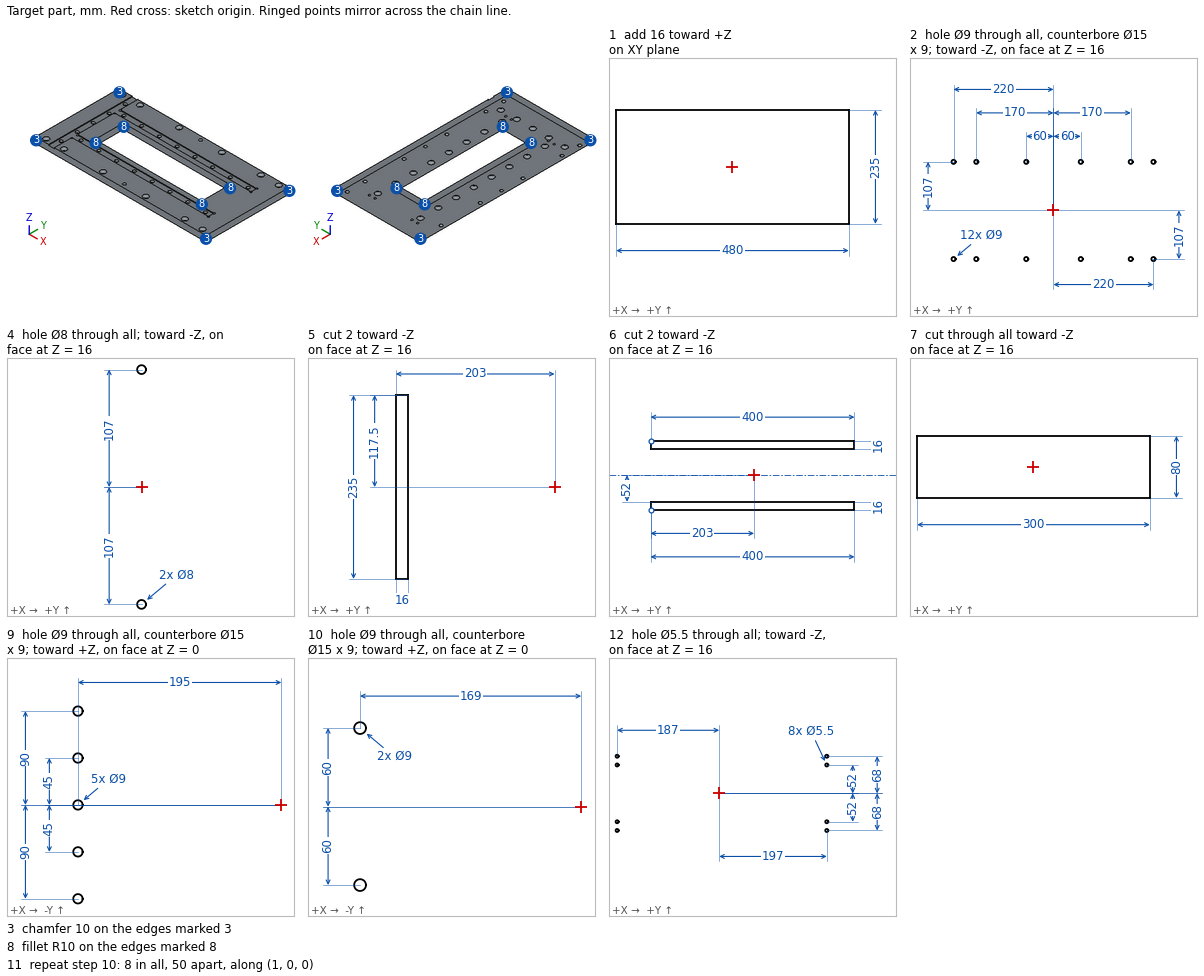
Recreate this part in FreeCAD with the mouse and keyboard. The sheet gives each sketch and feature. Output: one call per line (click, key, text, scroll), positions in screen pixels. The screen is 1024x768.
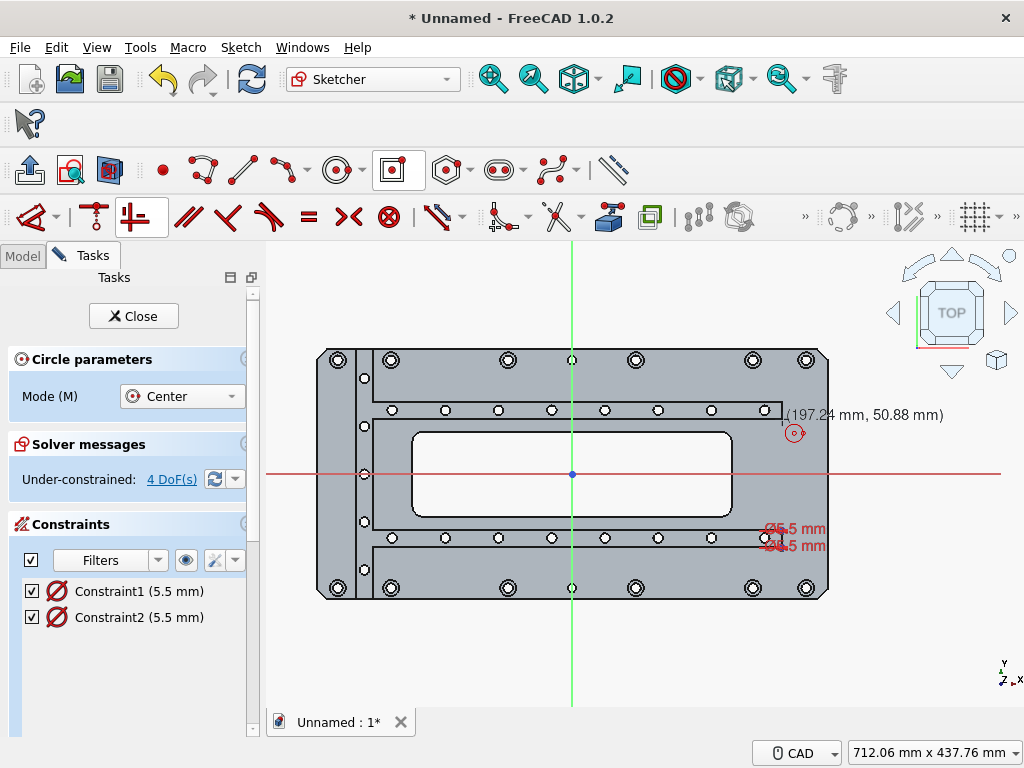
click(782, 419)
move(784, 417)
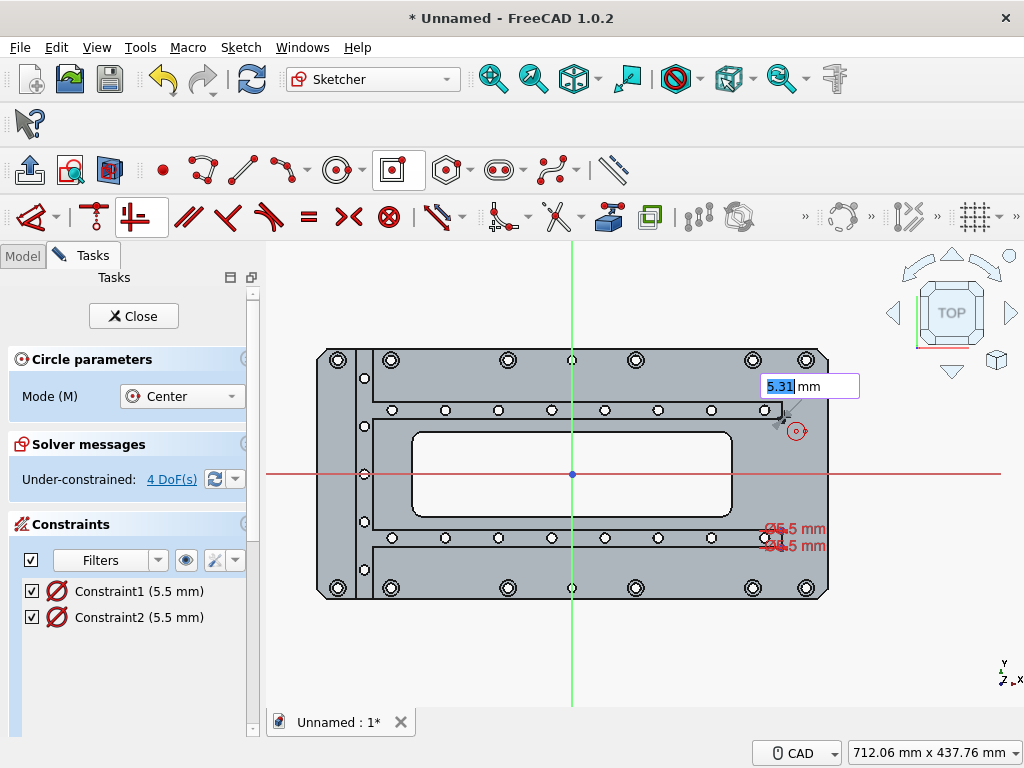
text(5.5)
key(Return)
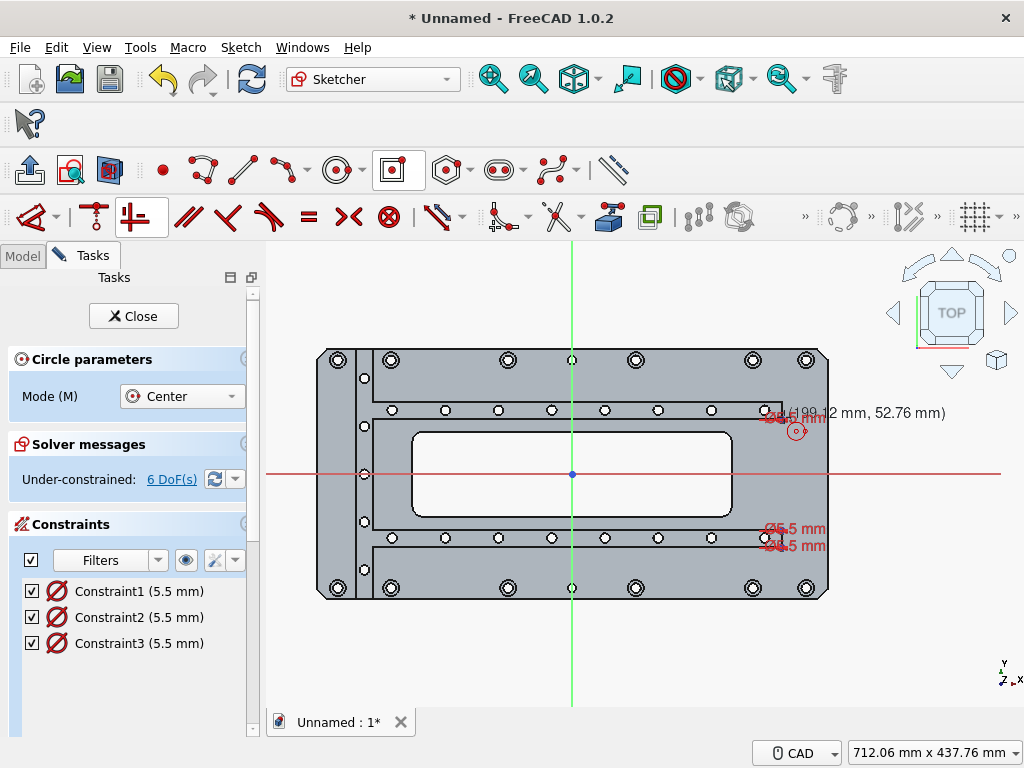
scroll(782, 402, up, 11)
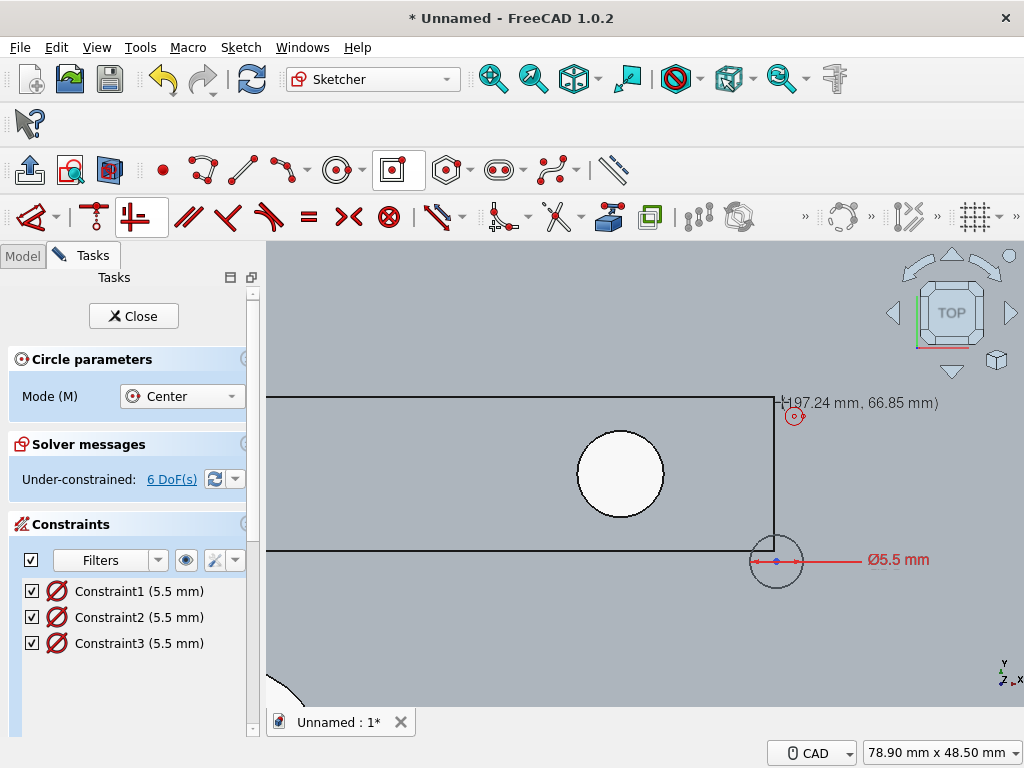
scroll(782, 402, down, 11)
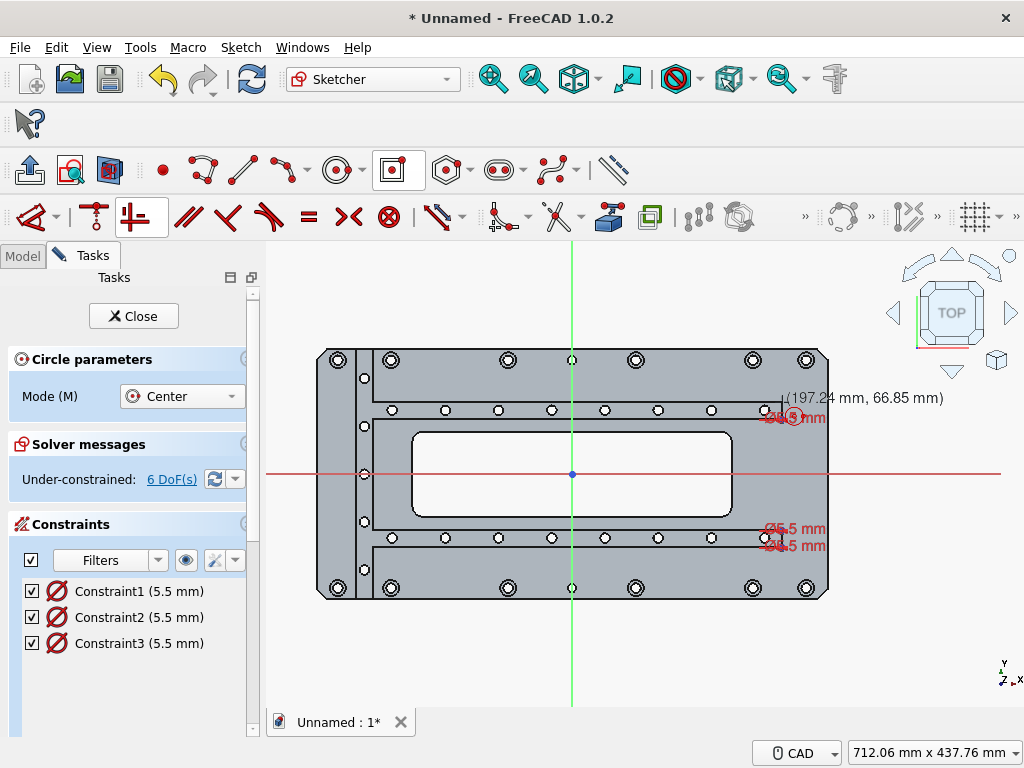
click(782, 402)
move(784, 400)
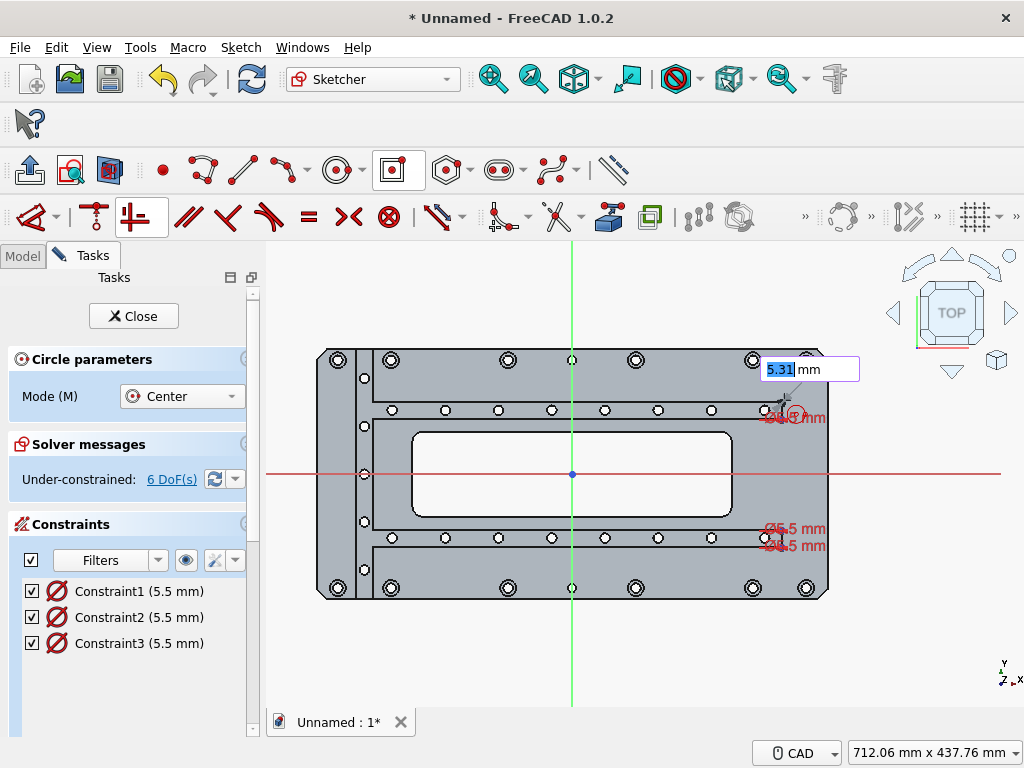
text(5.5)
key(Return)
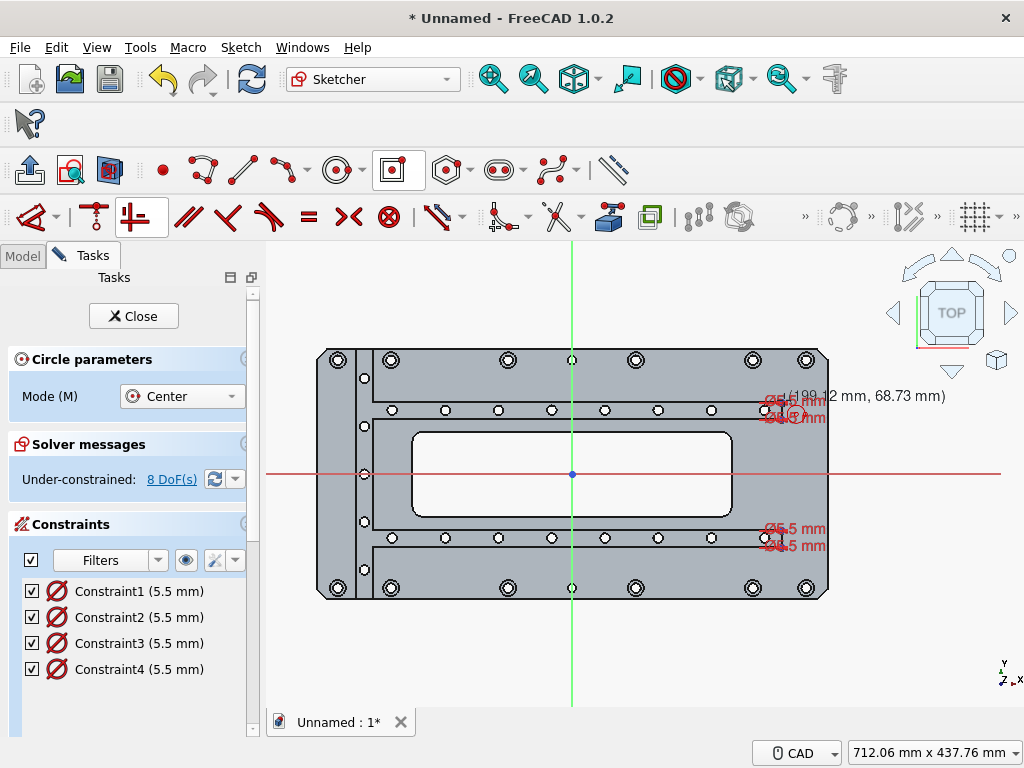
scroll(373, 402, up, 11)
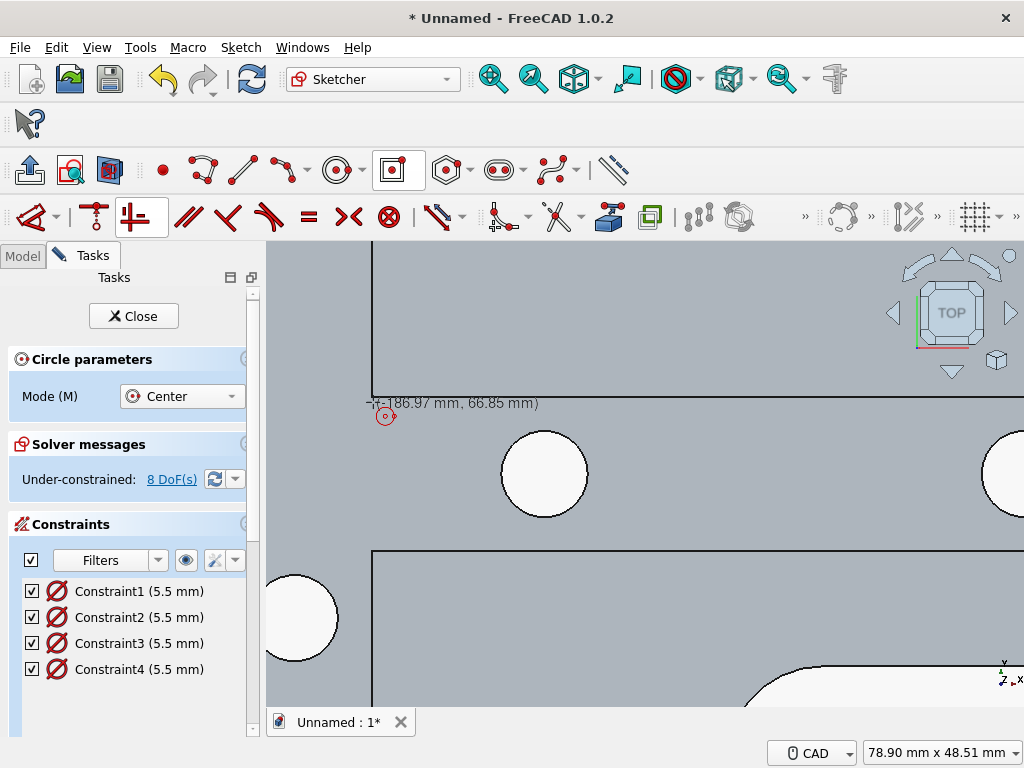
scroll(372, 402, down, 11)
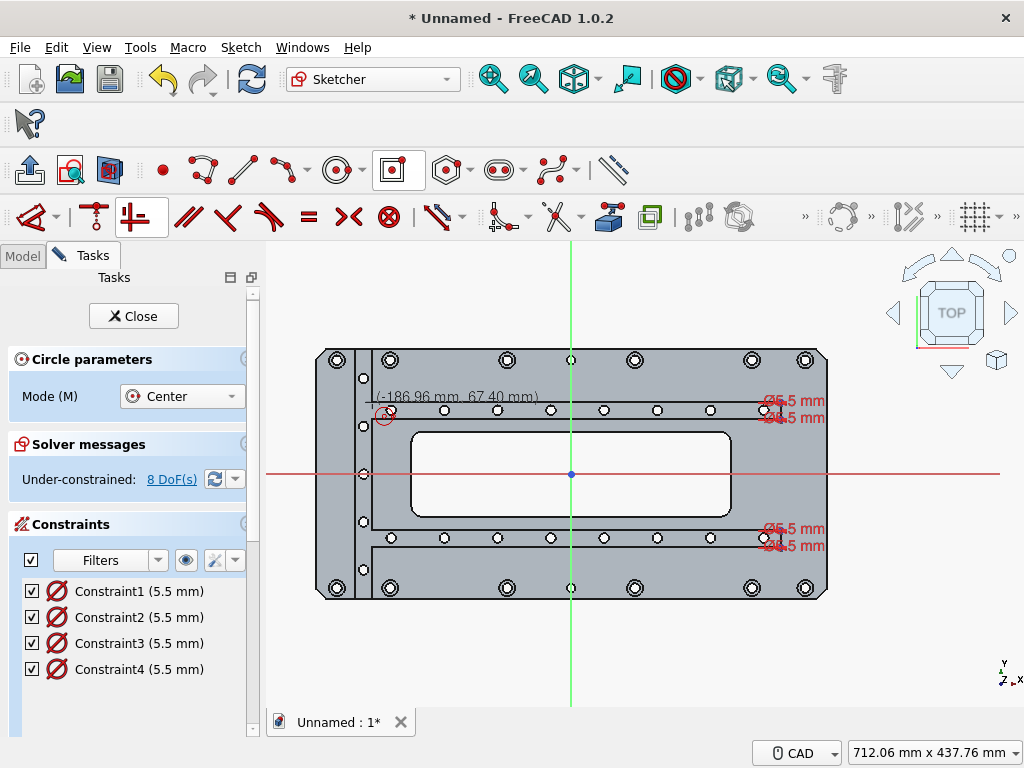
click(372, 402)
move(374, 400)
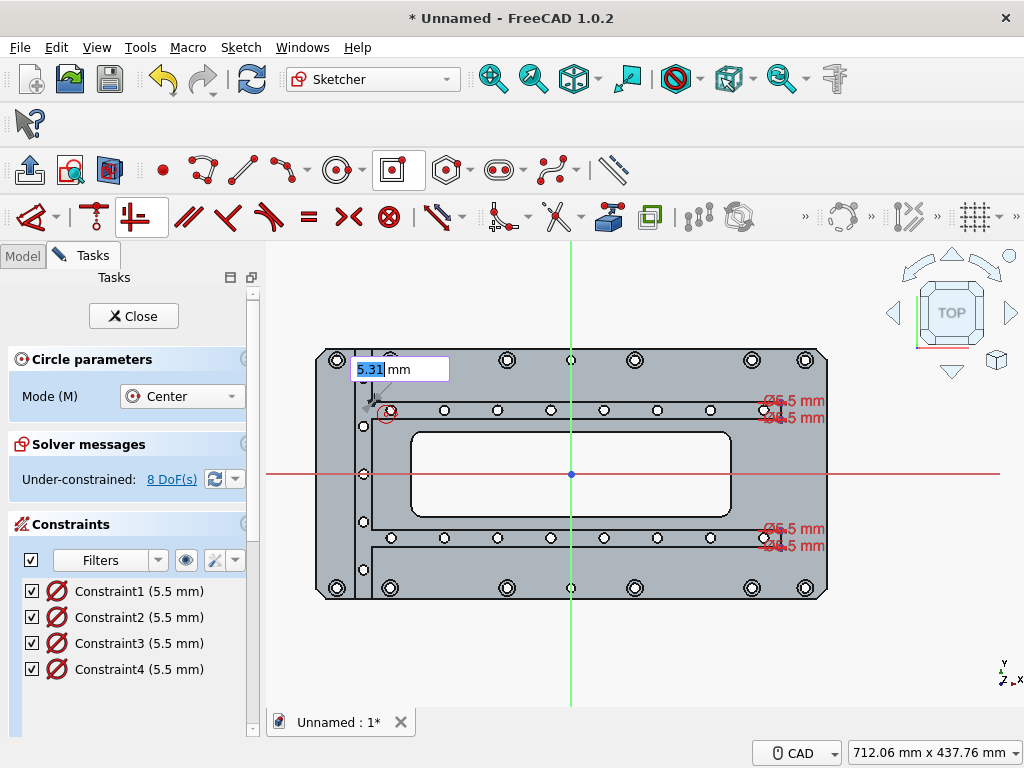
text(5.5)
key(Return)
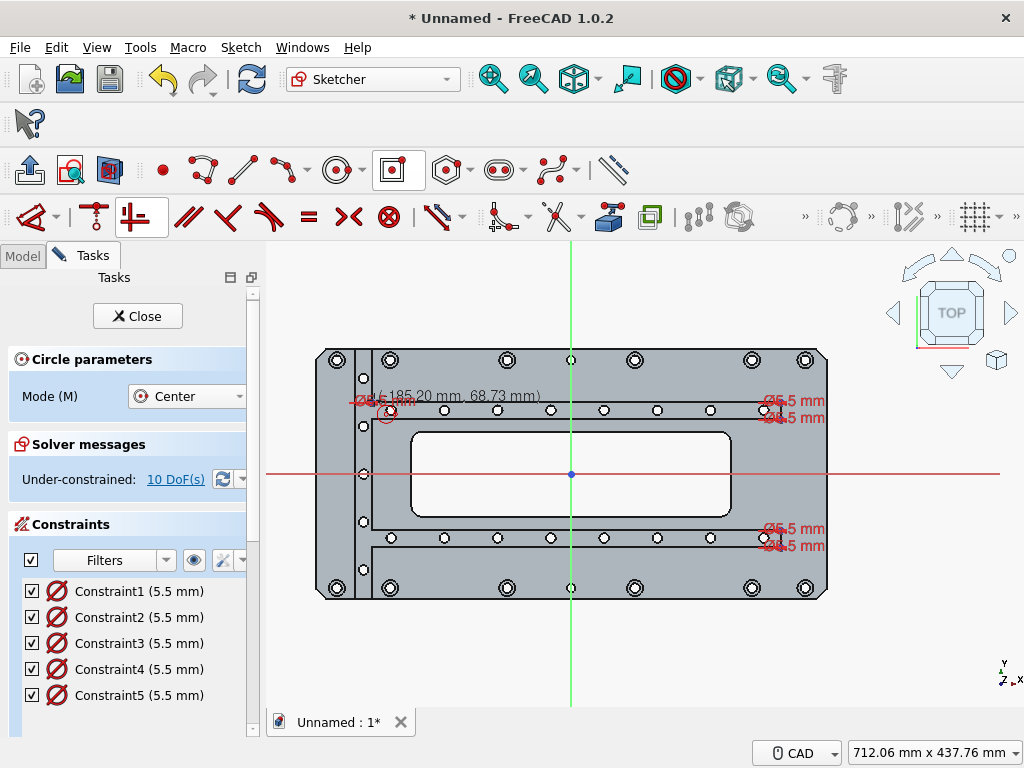
scroll(372, 419, up, 11)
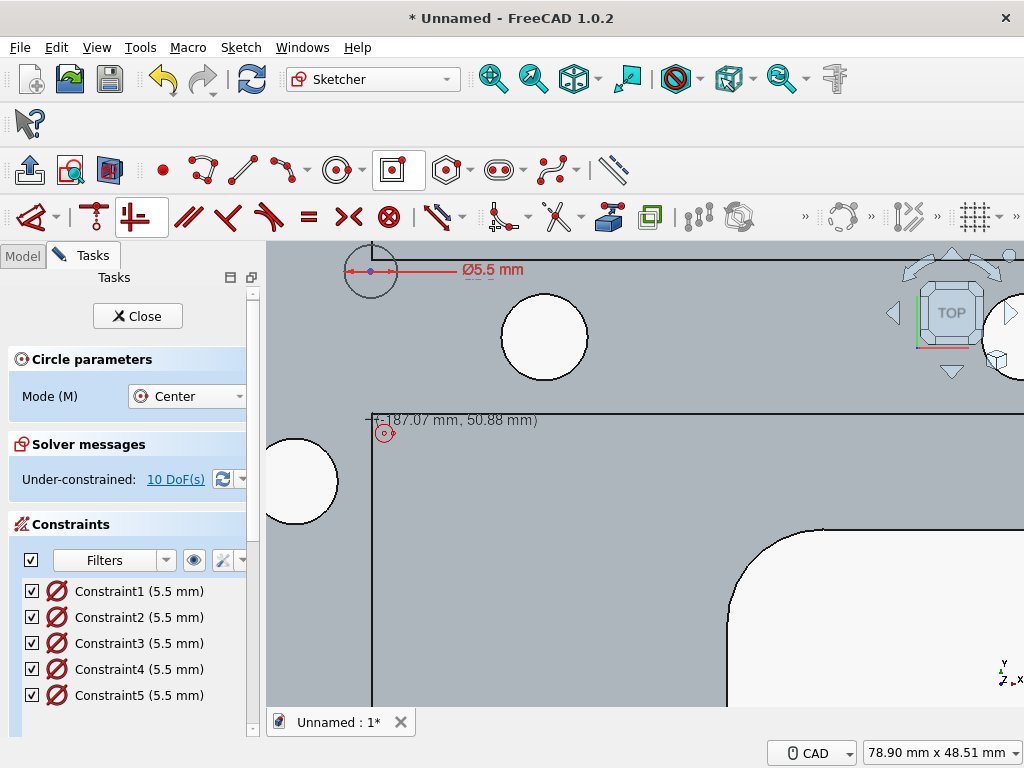
scroll(372, 419, down, 11)